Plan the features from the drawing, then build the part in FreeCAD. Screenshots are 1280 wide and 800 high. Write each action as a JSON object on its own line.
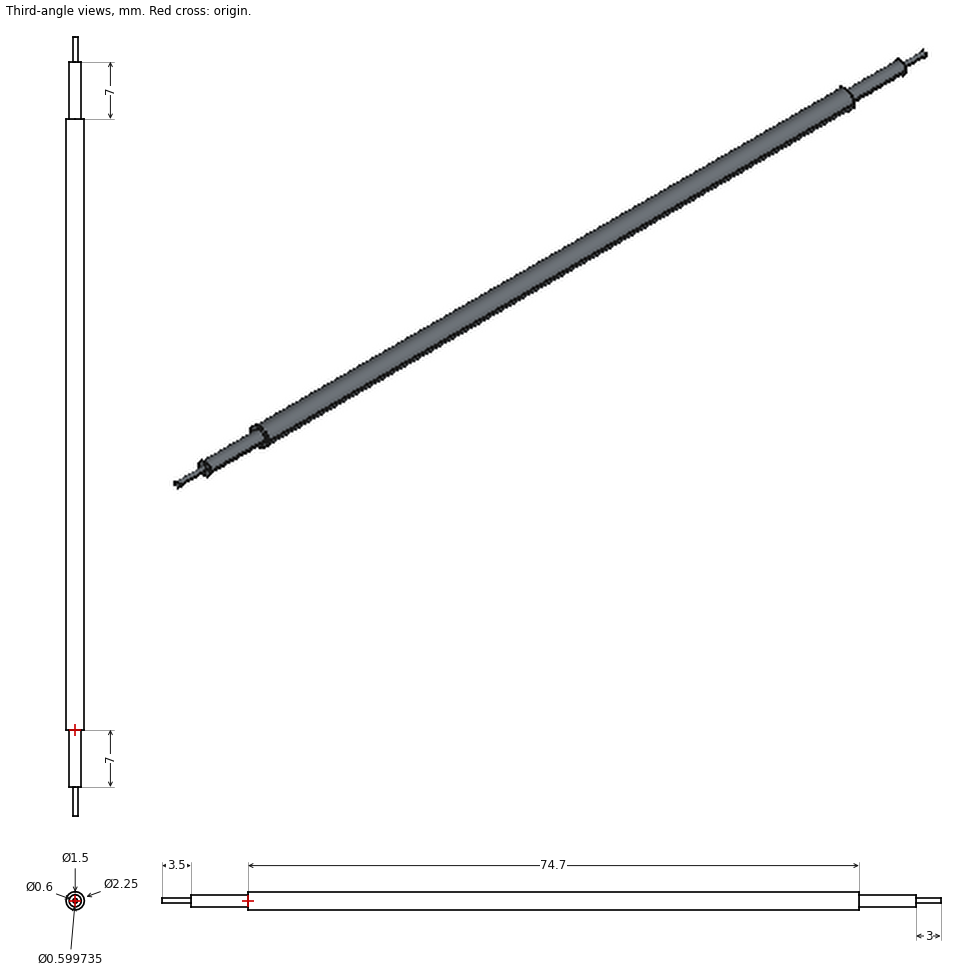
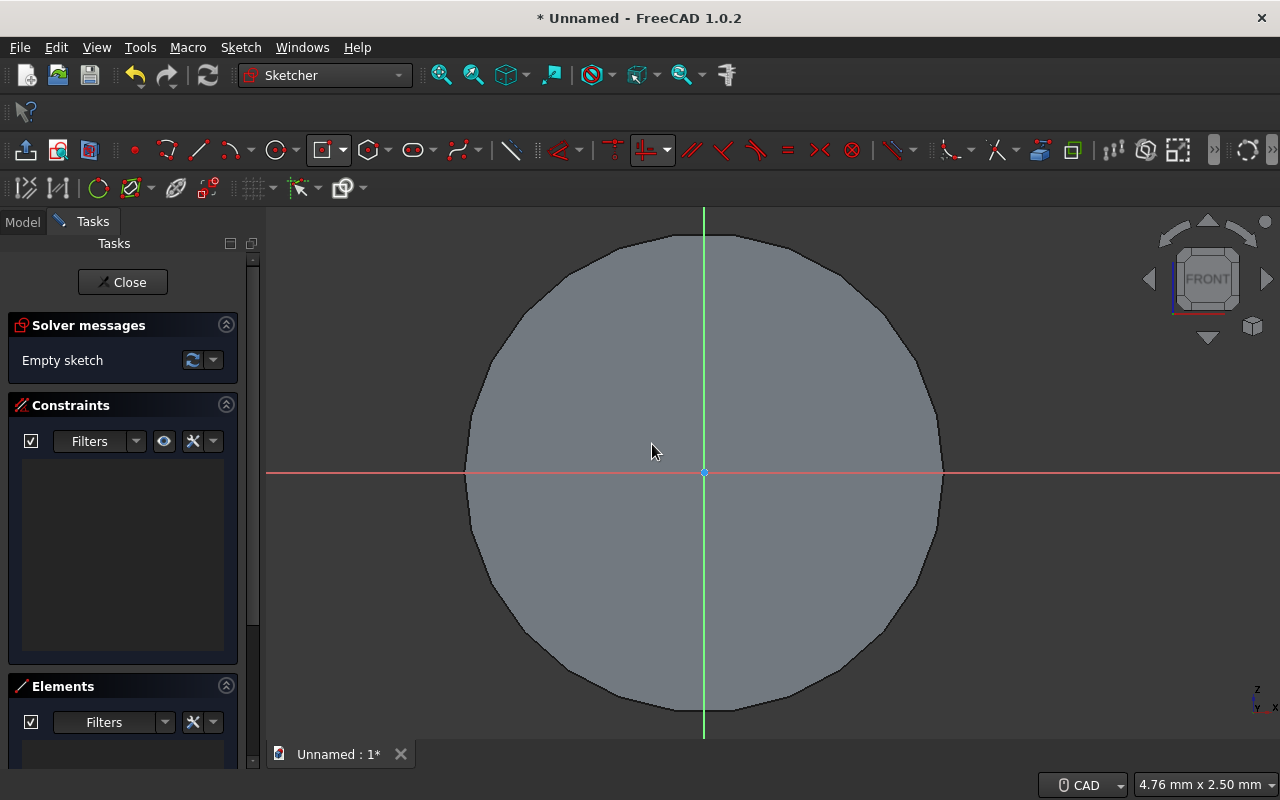
{"action": "left_click", "coordinate": [276, 150]}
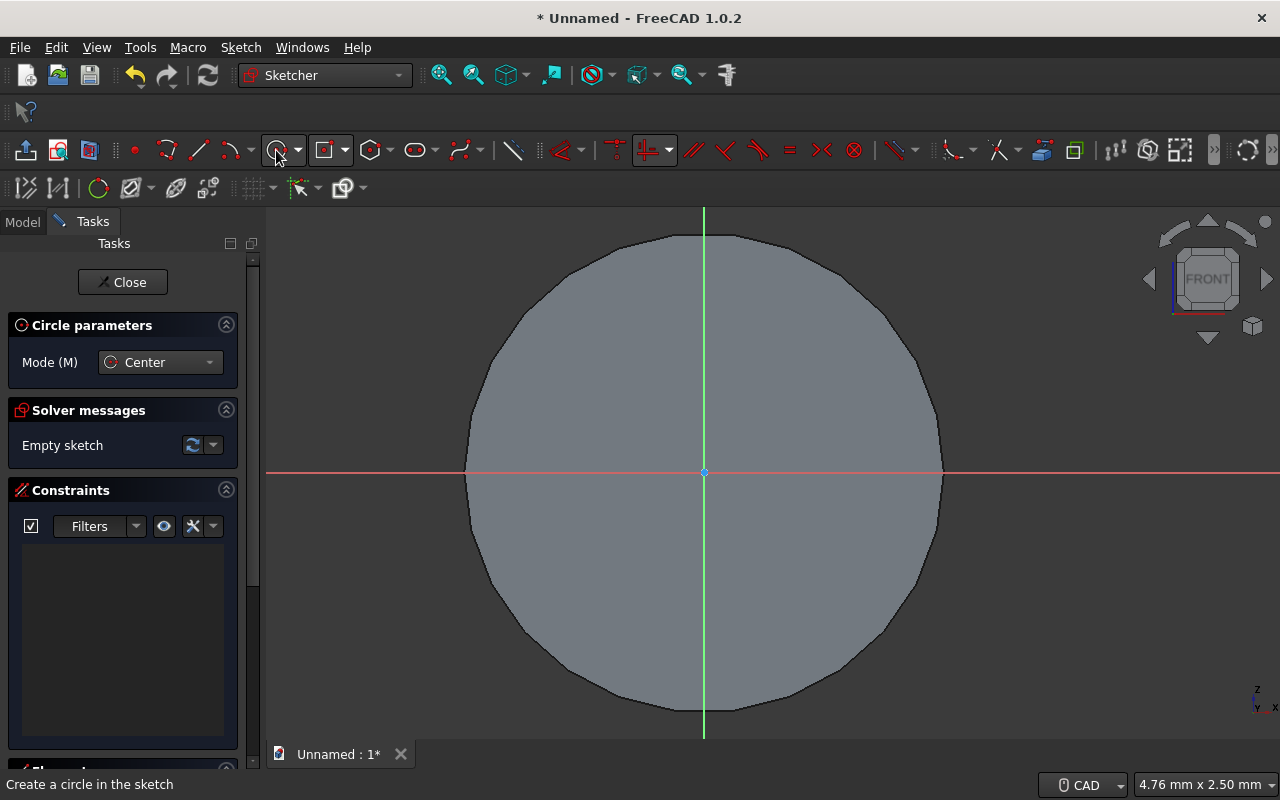
{"action": "left_click", "coordinate": [704, 473]}
{"action": "mouse_move", "coordinate": [817, 360]}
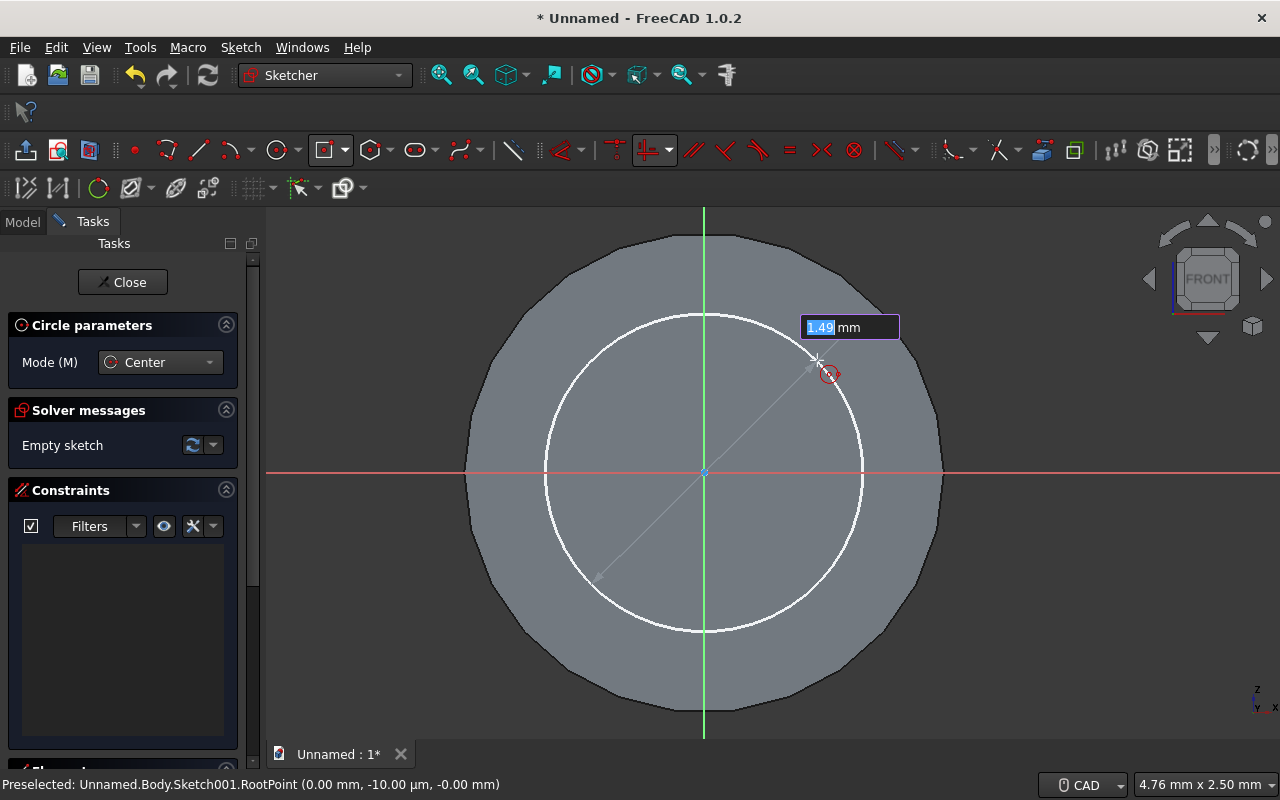
{"action": "type", "text": "1.5"}
{"action": "key", "text": "Return"}
{"action": "key", "text": "Escape"}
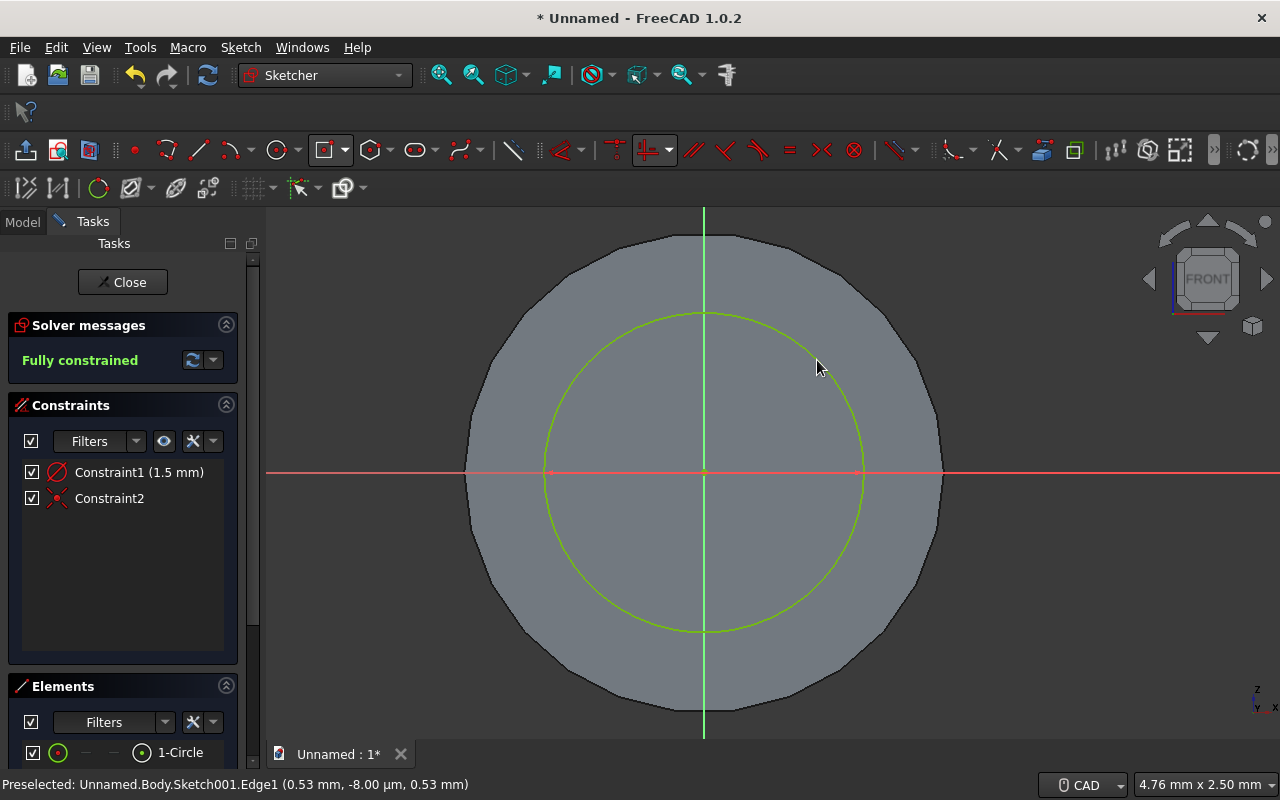
{"action": "left_click", "coordinate": [123, 282]}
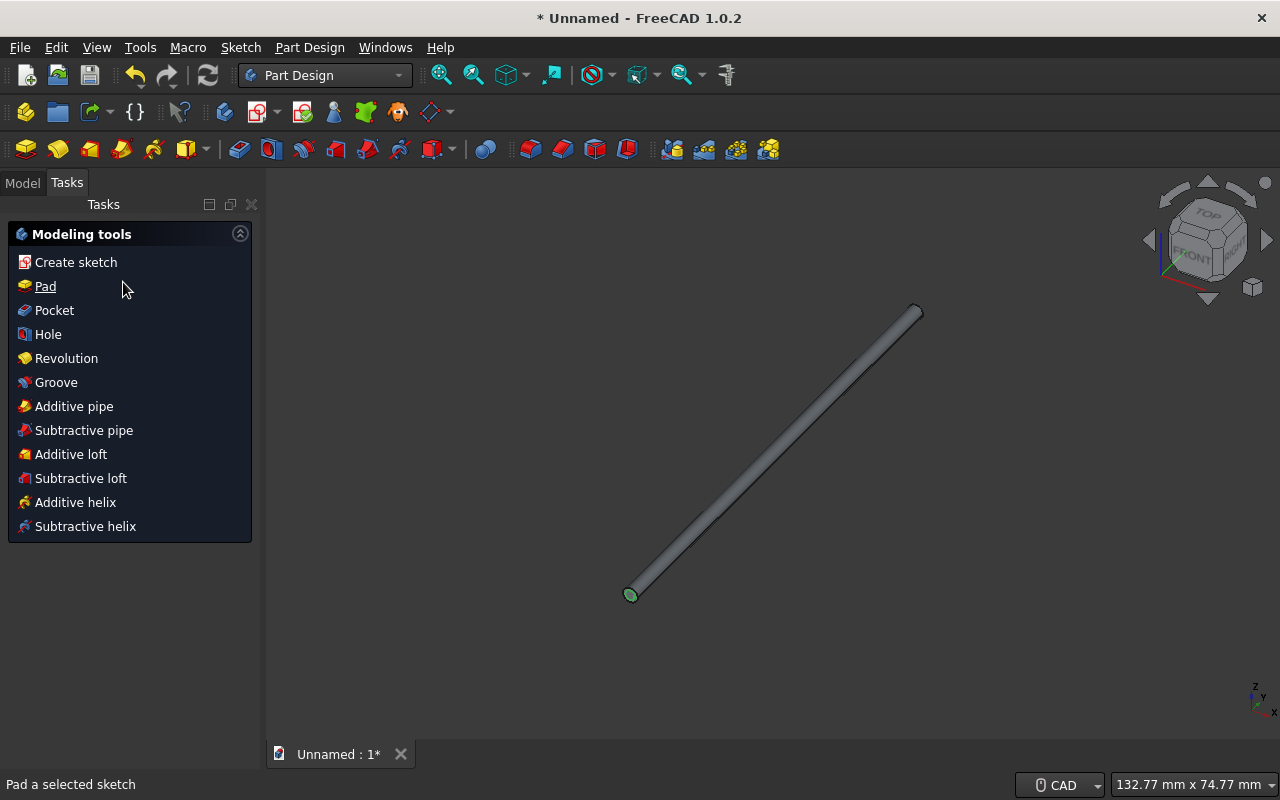
{"action": "left_click", "coordinate": [26, 150]}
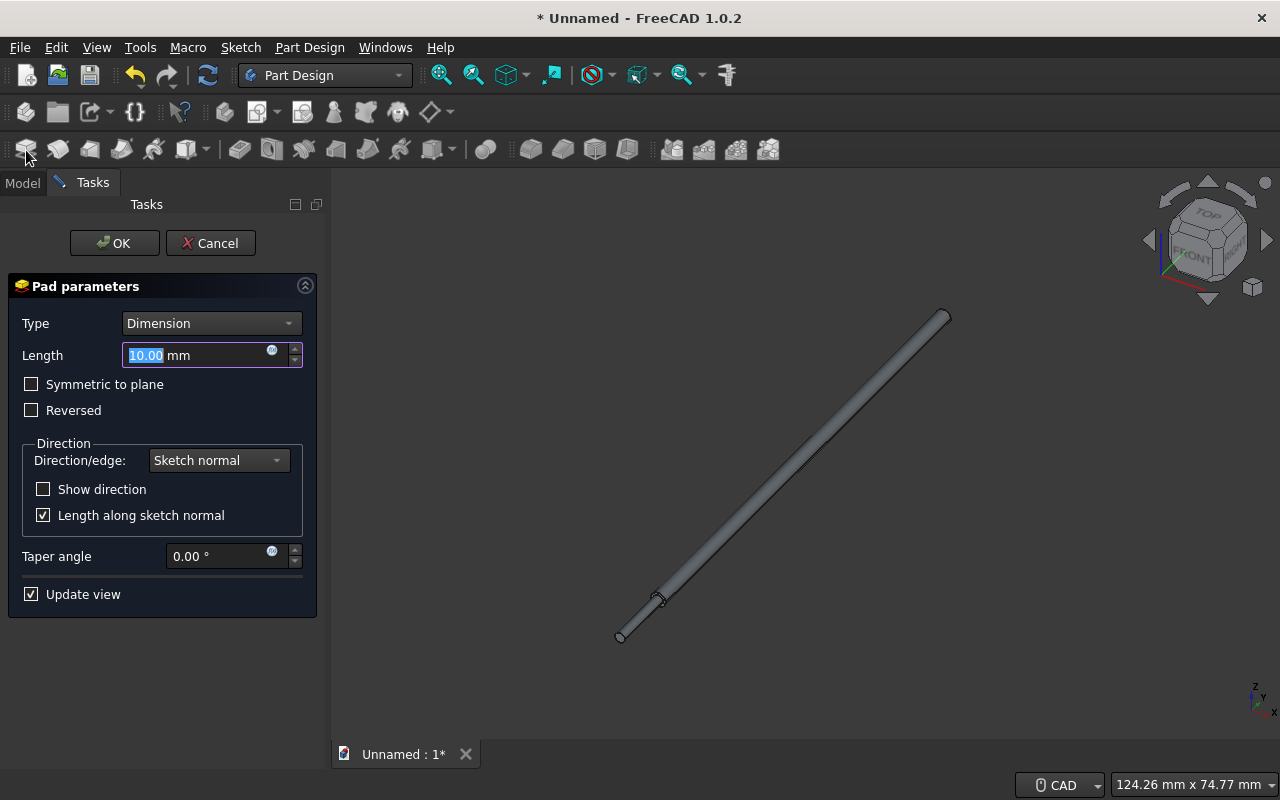
{"action": "type", "text": "7"}
{"action": "key", "text": "Tab"}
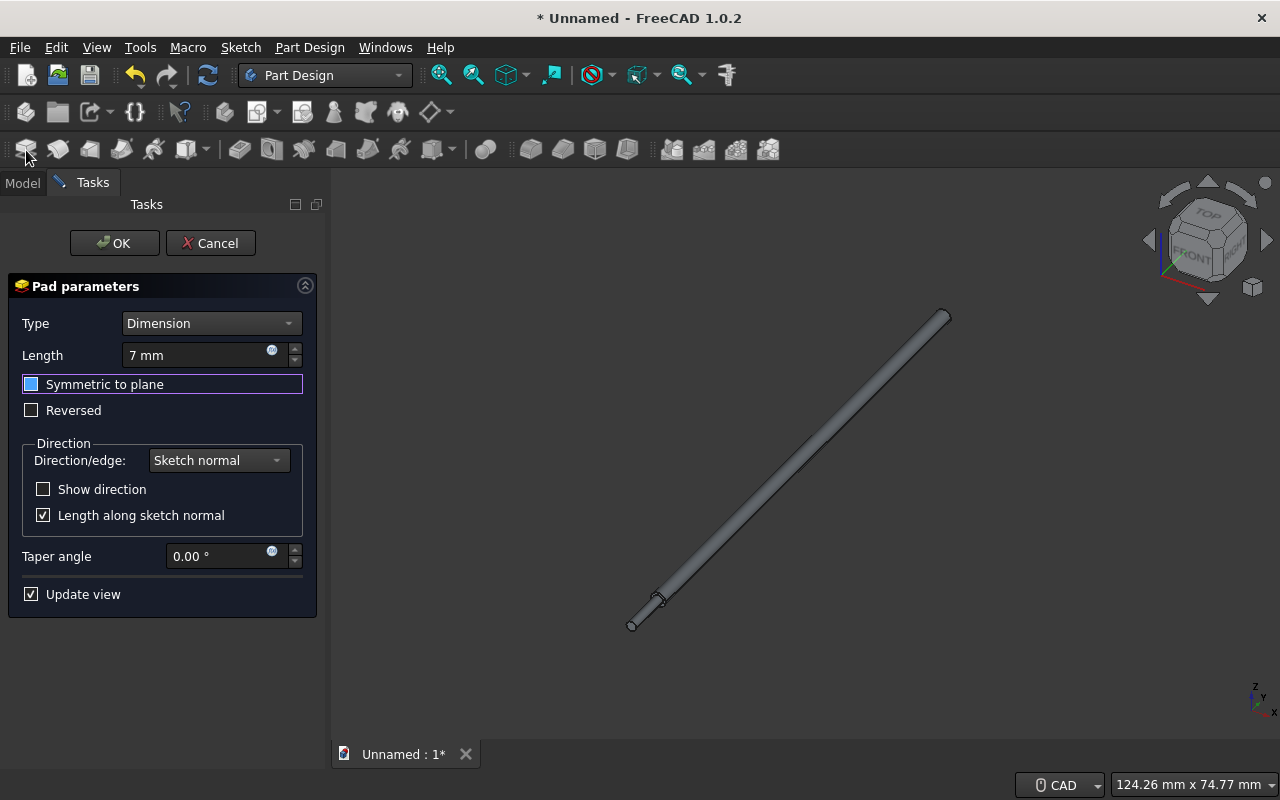
{"action": "left_click", "coordinate": [115, 243]}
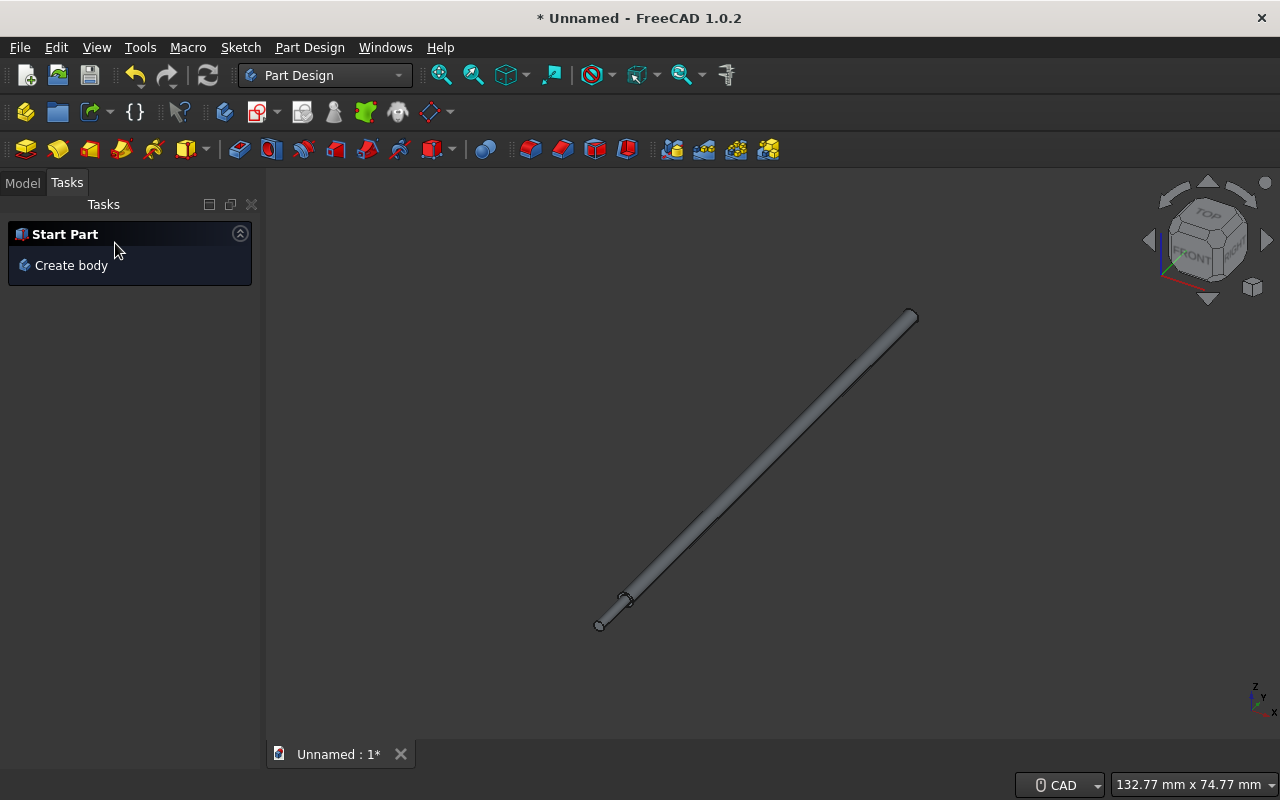
{"action": "scroll", "coordinate": [599, 625], "scroll_direction": "up", "scroll_amount": 4}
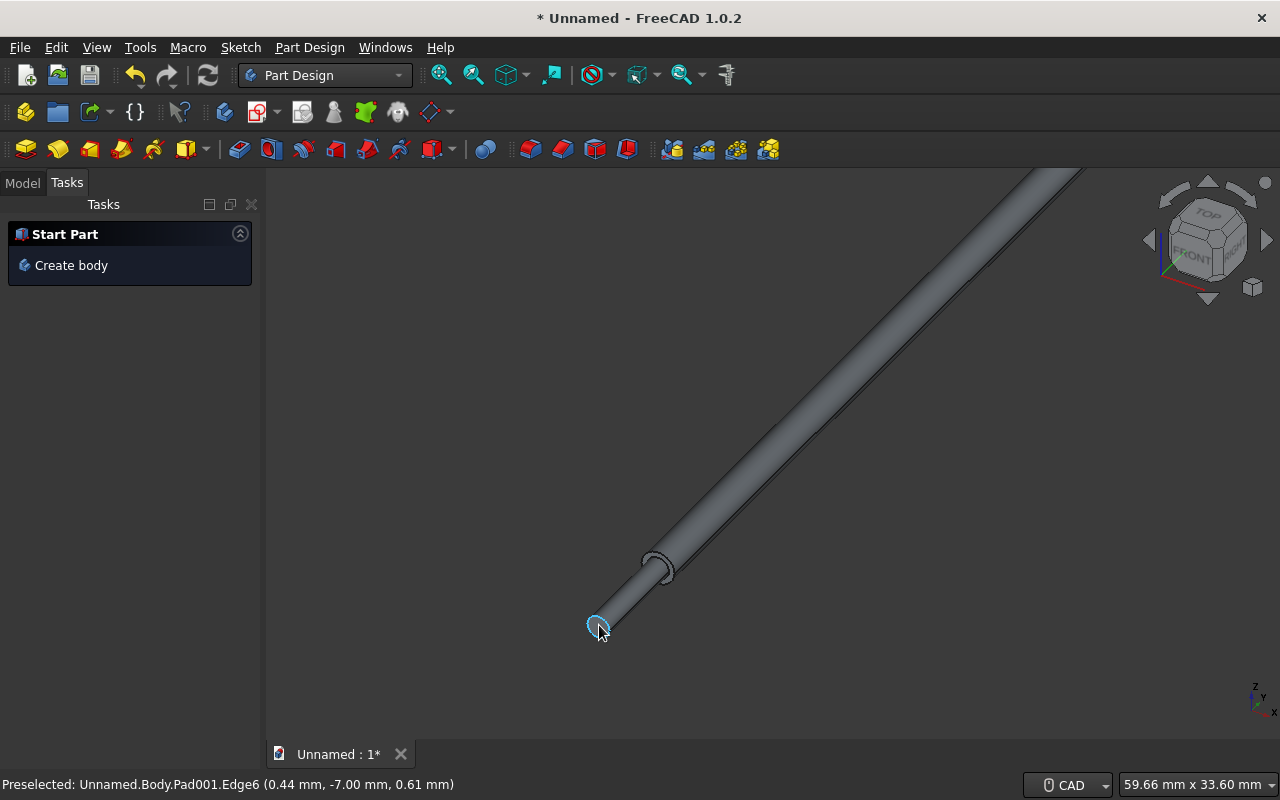
{"action": "left_click", "coordinate": [599, 629]}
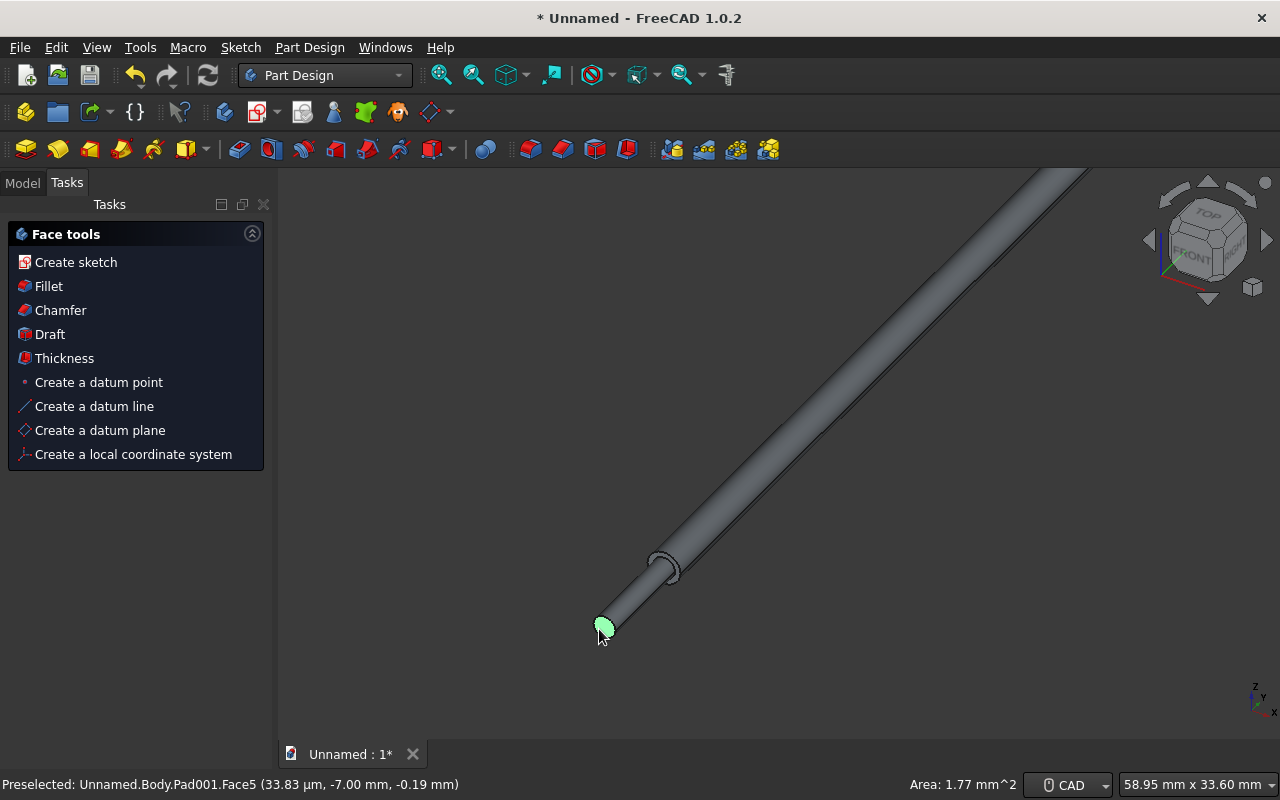
{"action": "left_click", "coordinate": [258, 112]}